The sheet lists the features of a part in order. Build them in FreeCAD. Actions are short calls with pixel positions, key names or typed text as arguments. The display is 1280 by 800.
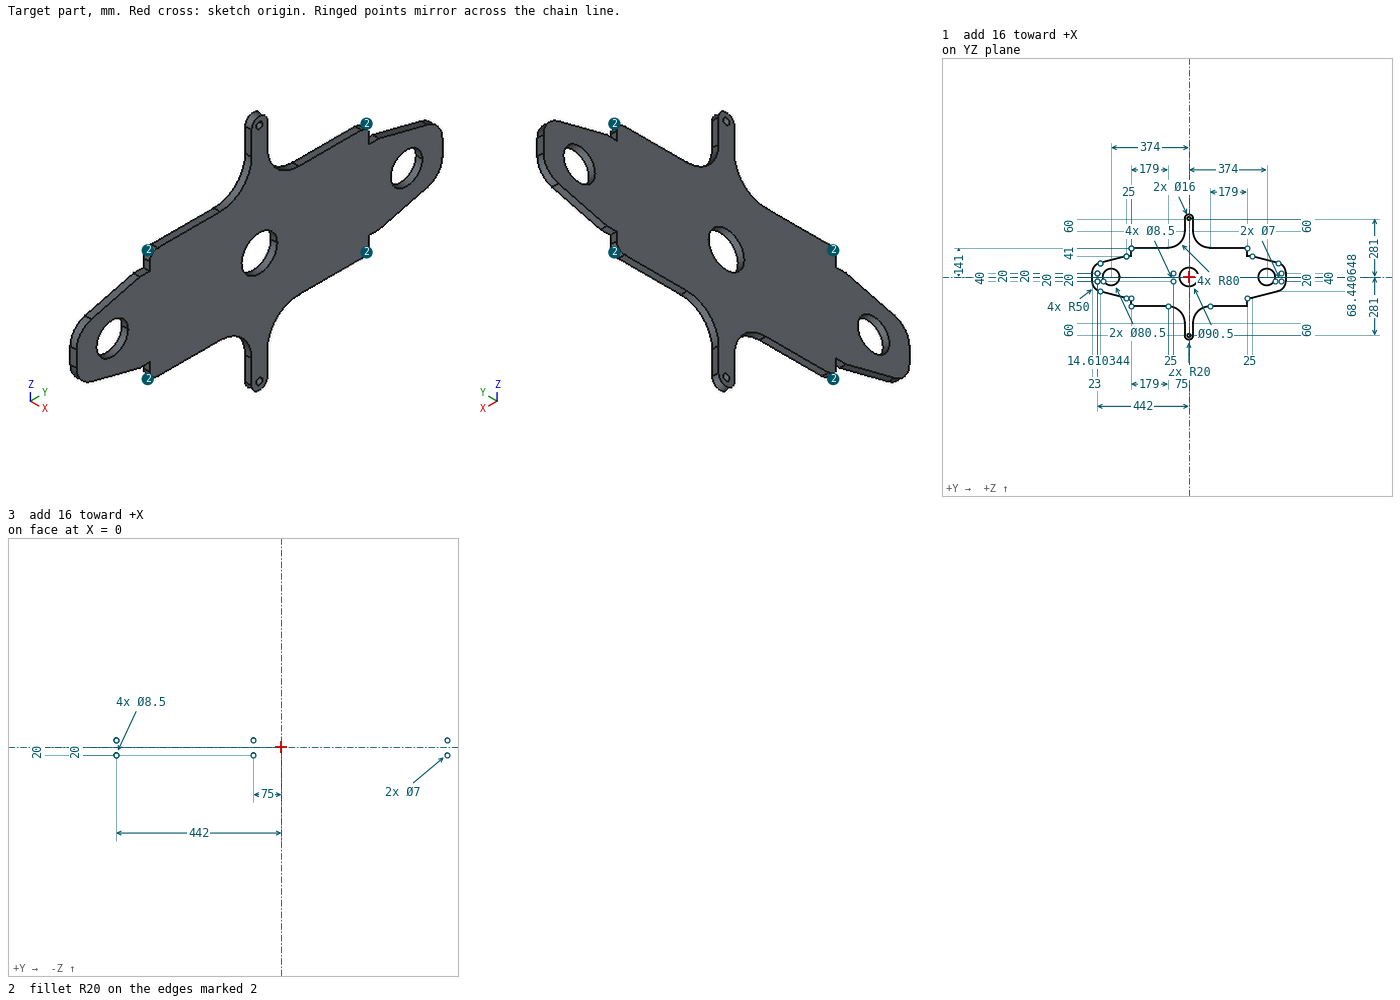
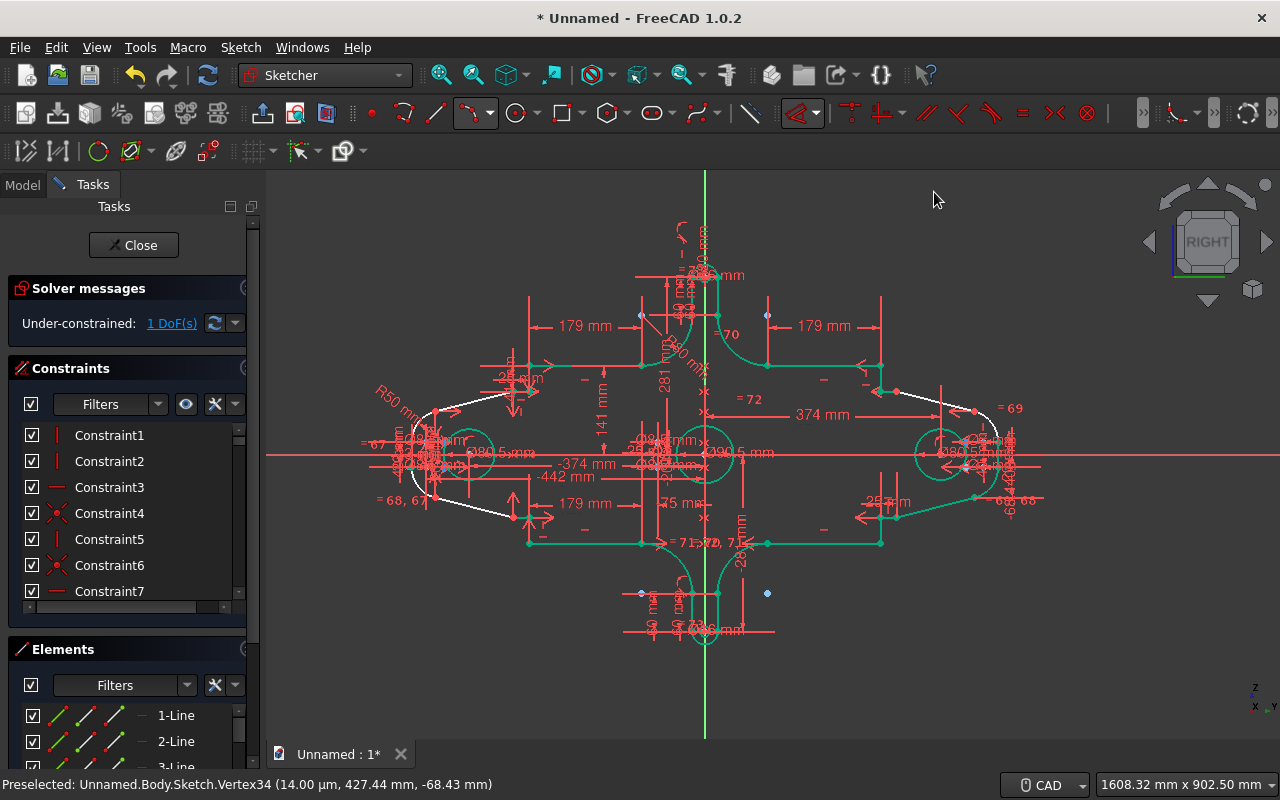
scroll(435, 498, up, 8)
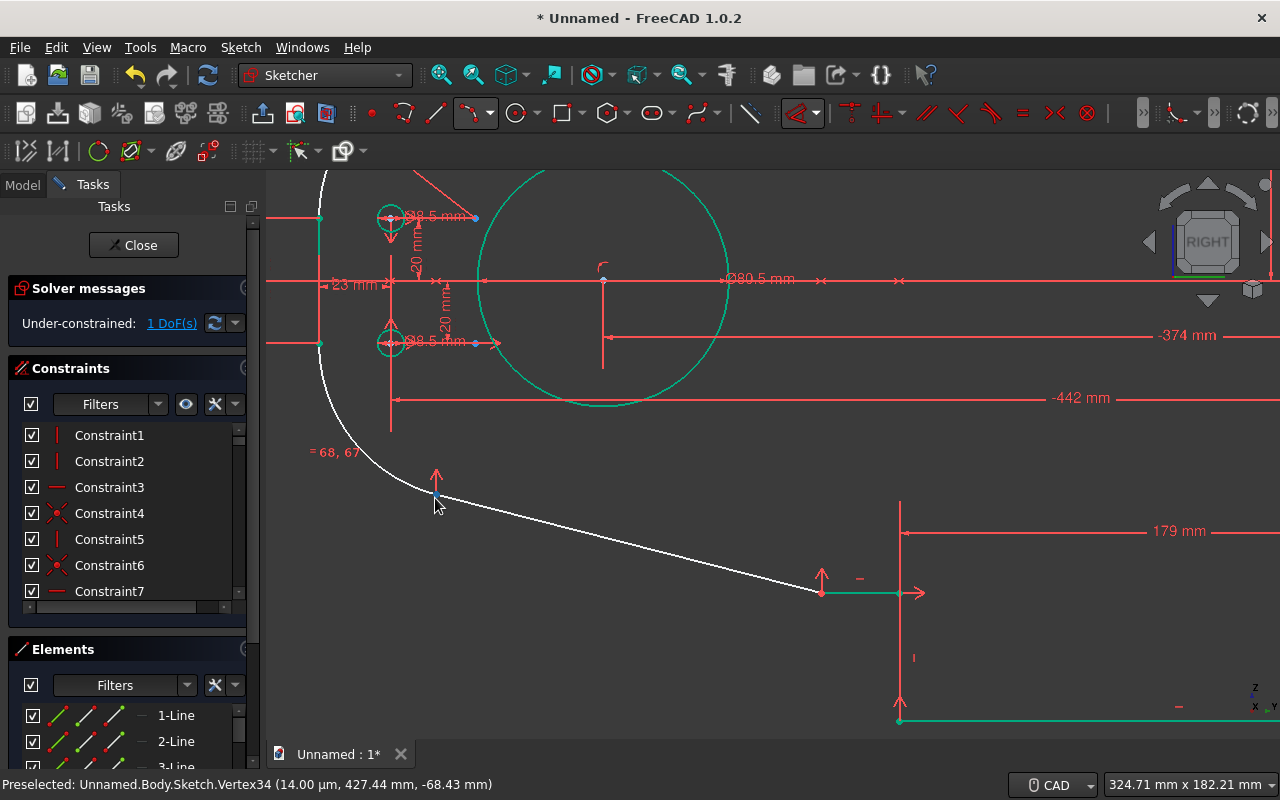
click(436, 495)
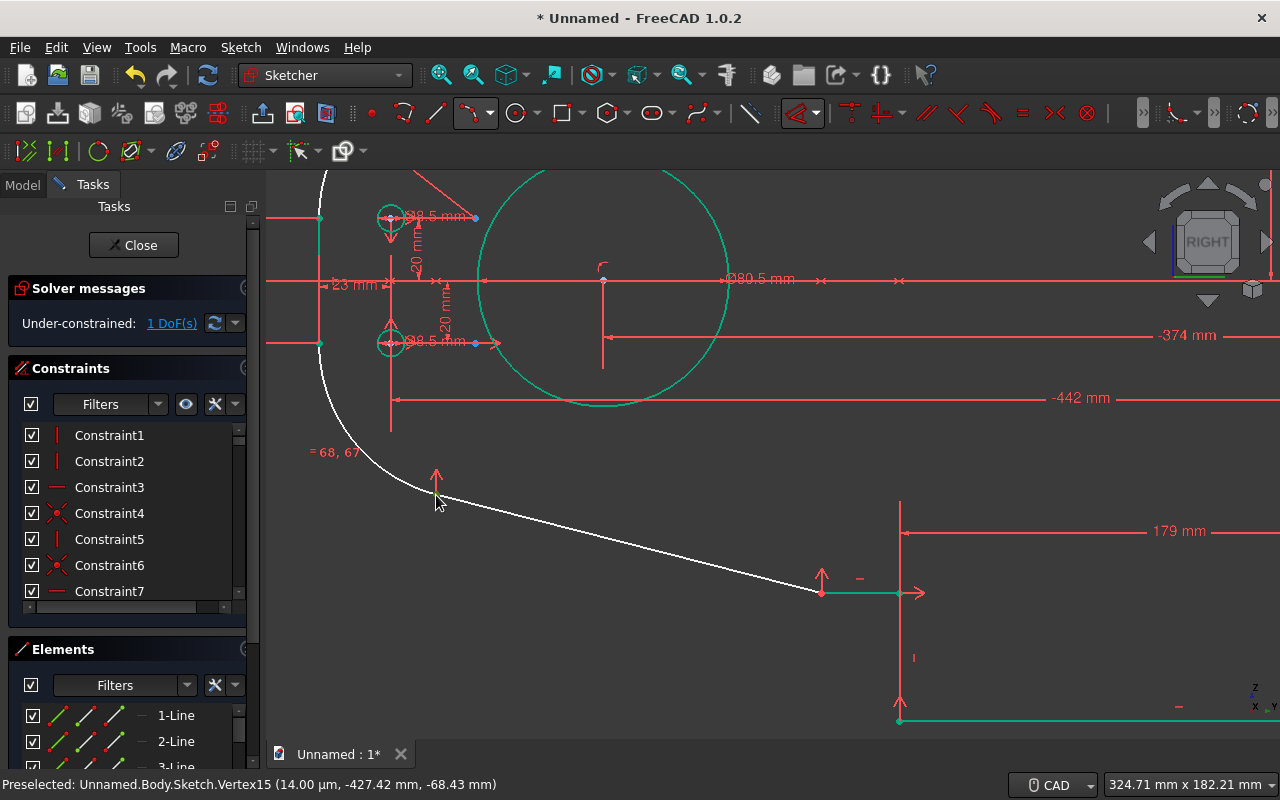
click(391, 343)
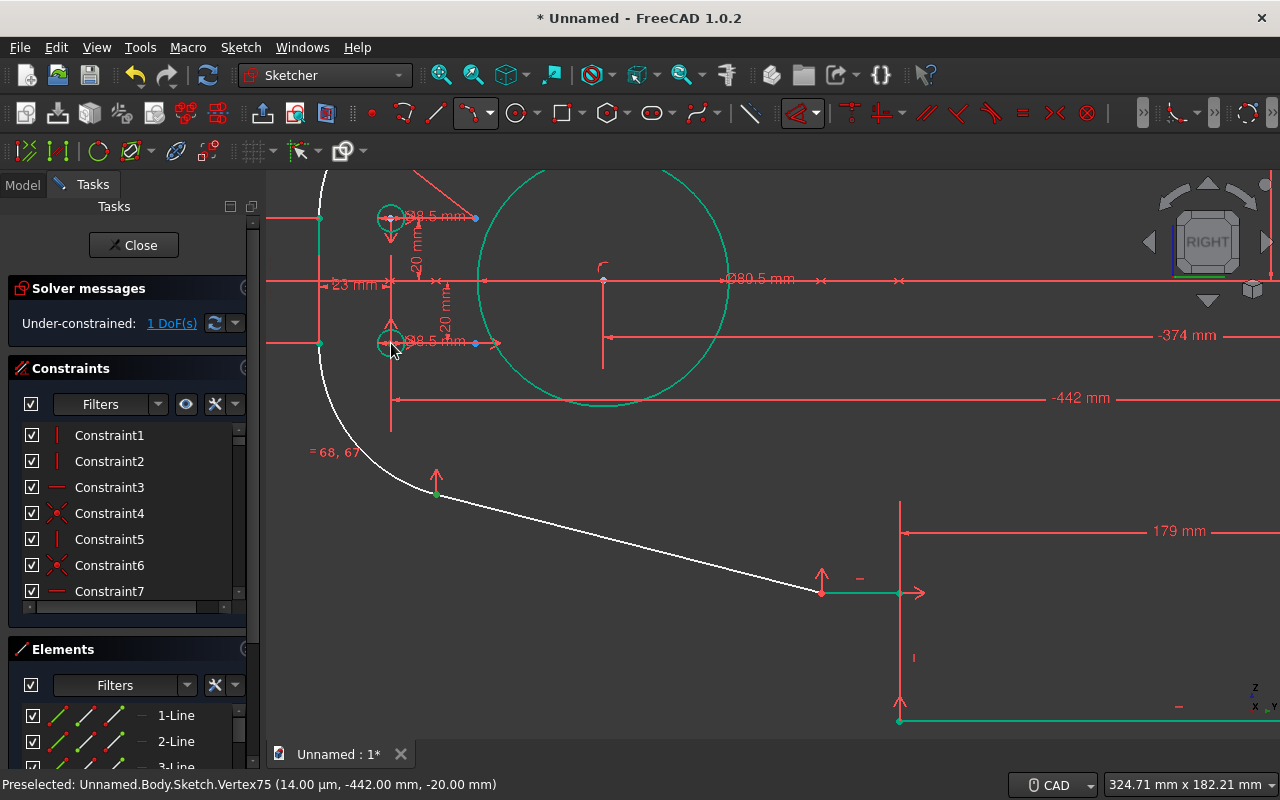
click(818, 114)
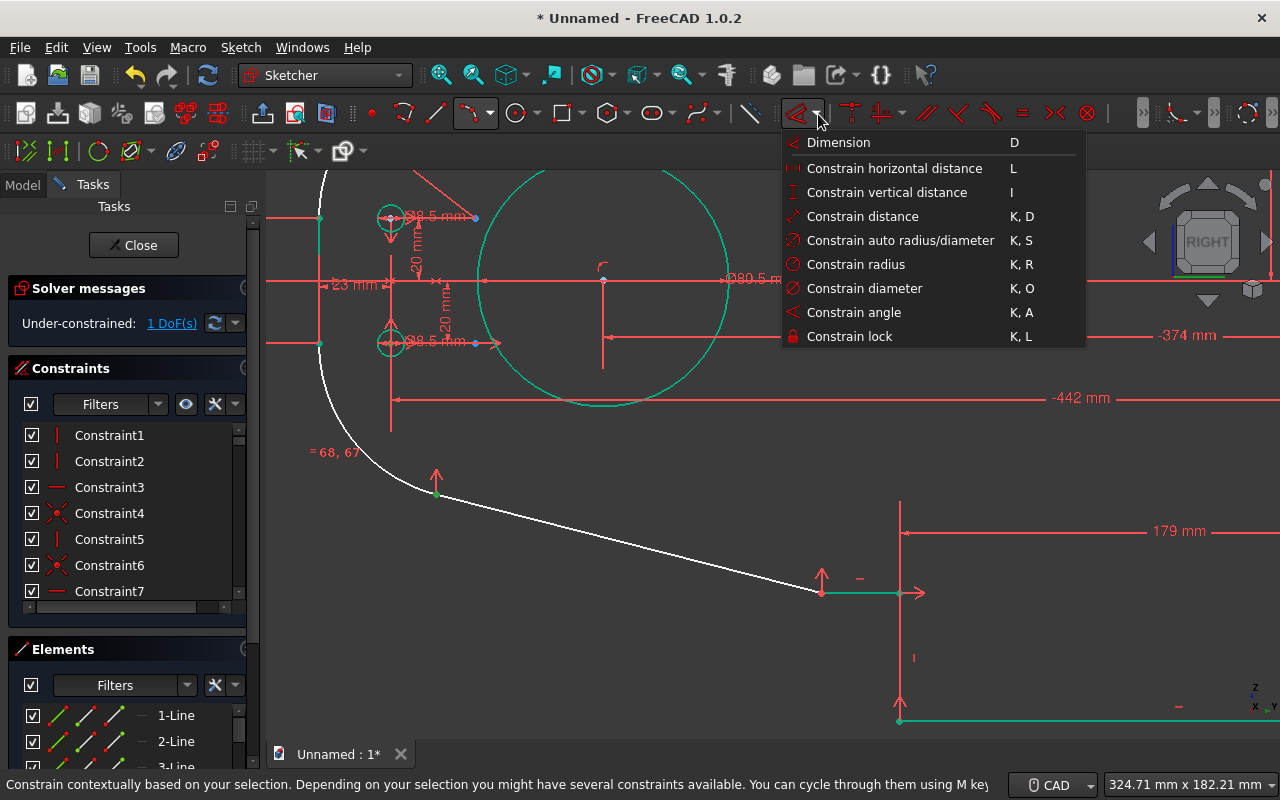
click(934, 168)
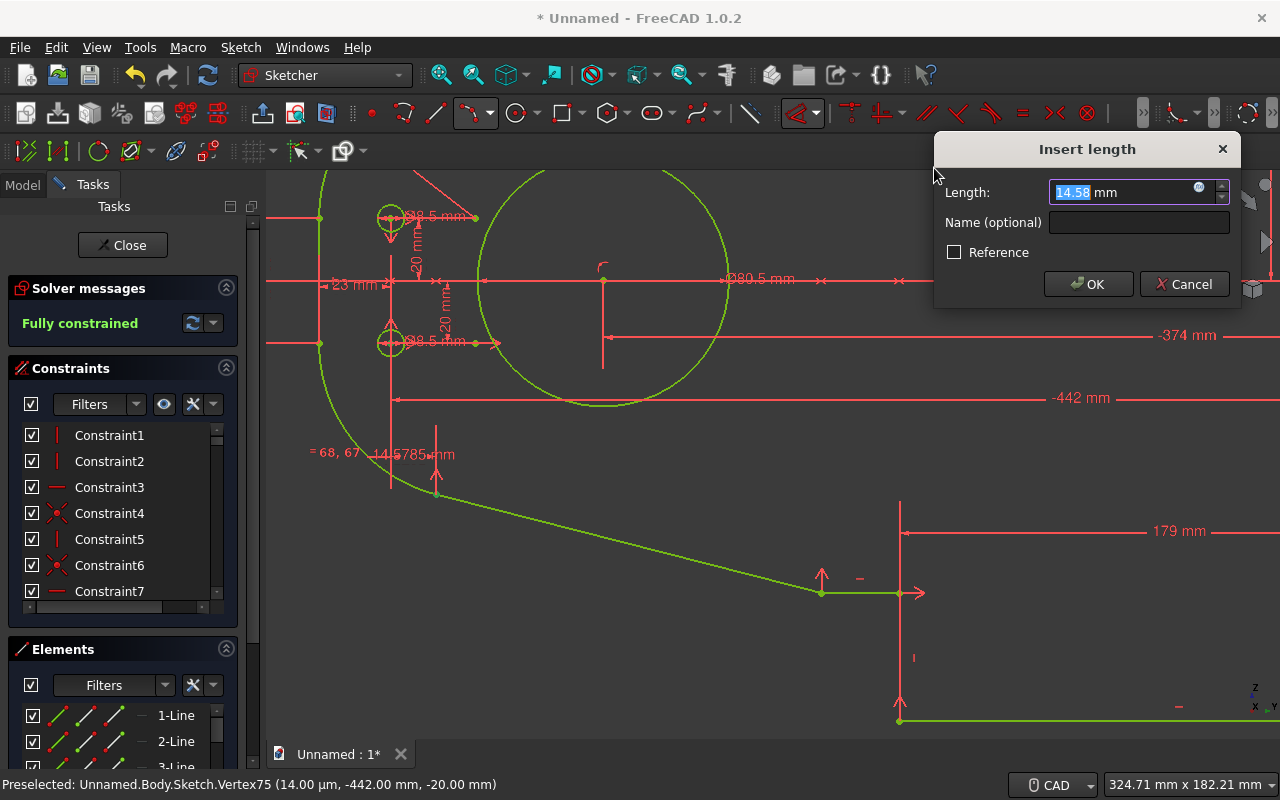
text(14.610344)
key(Return)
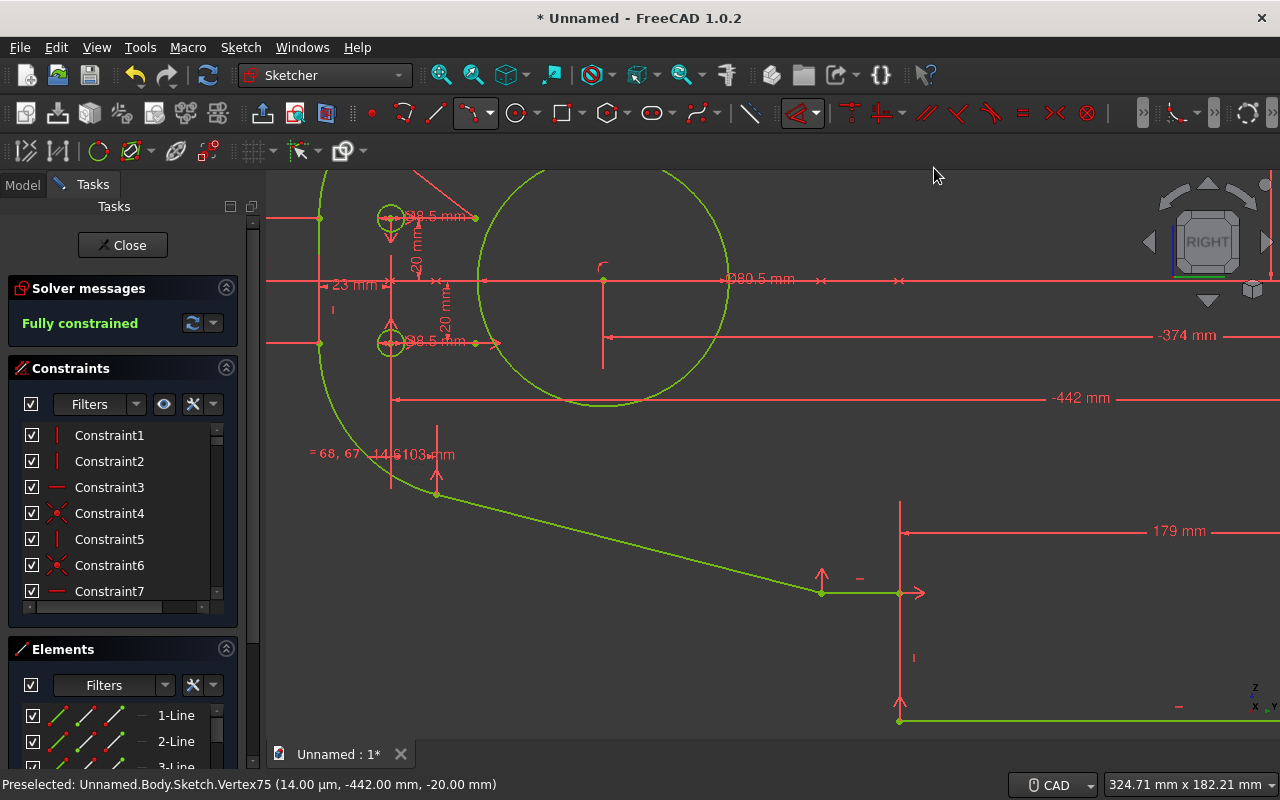
click(123, 245)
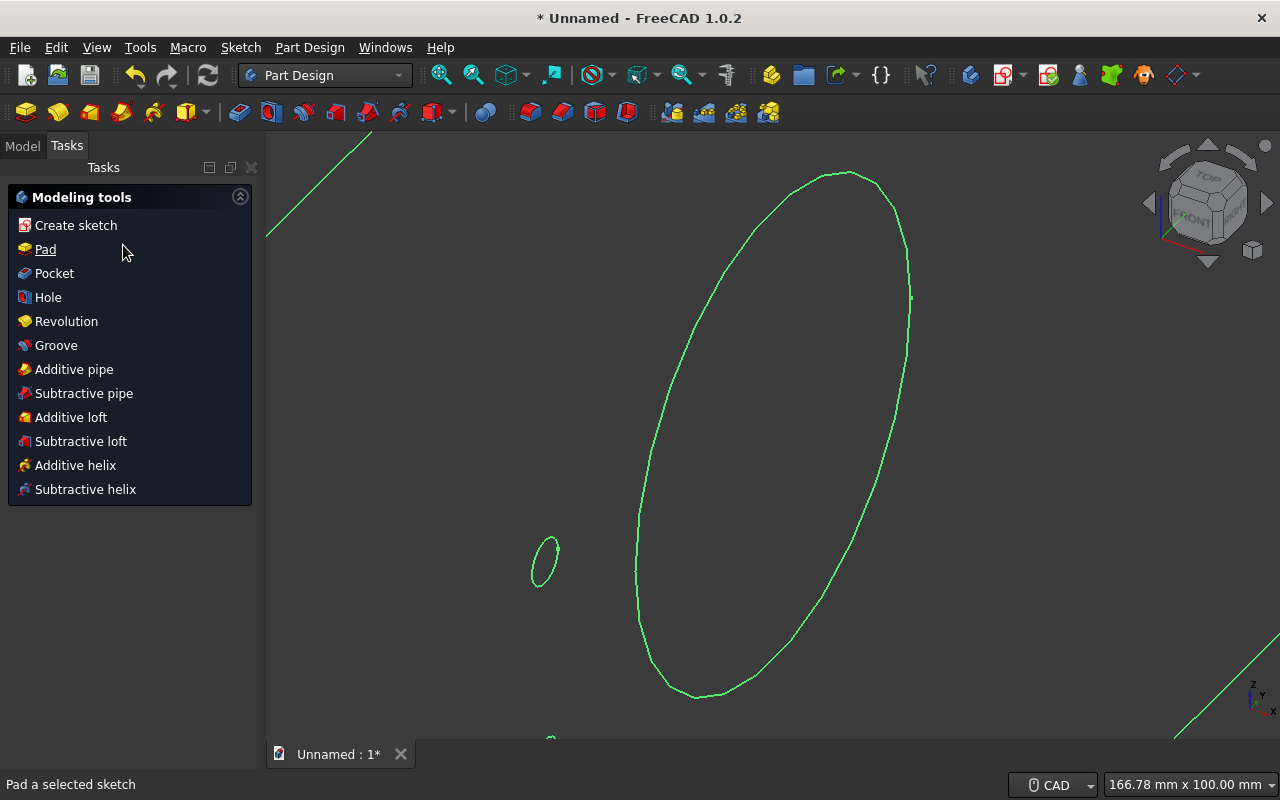
click(26, 112)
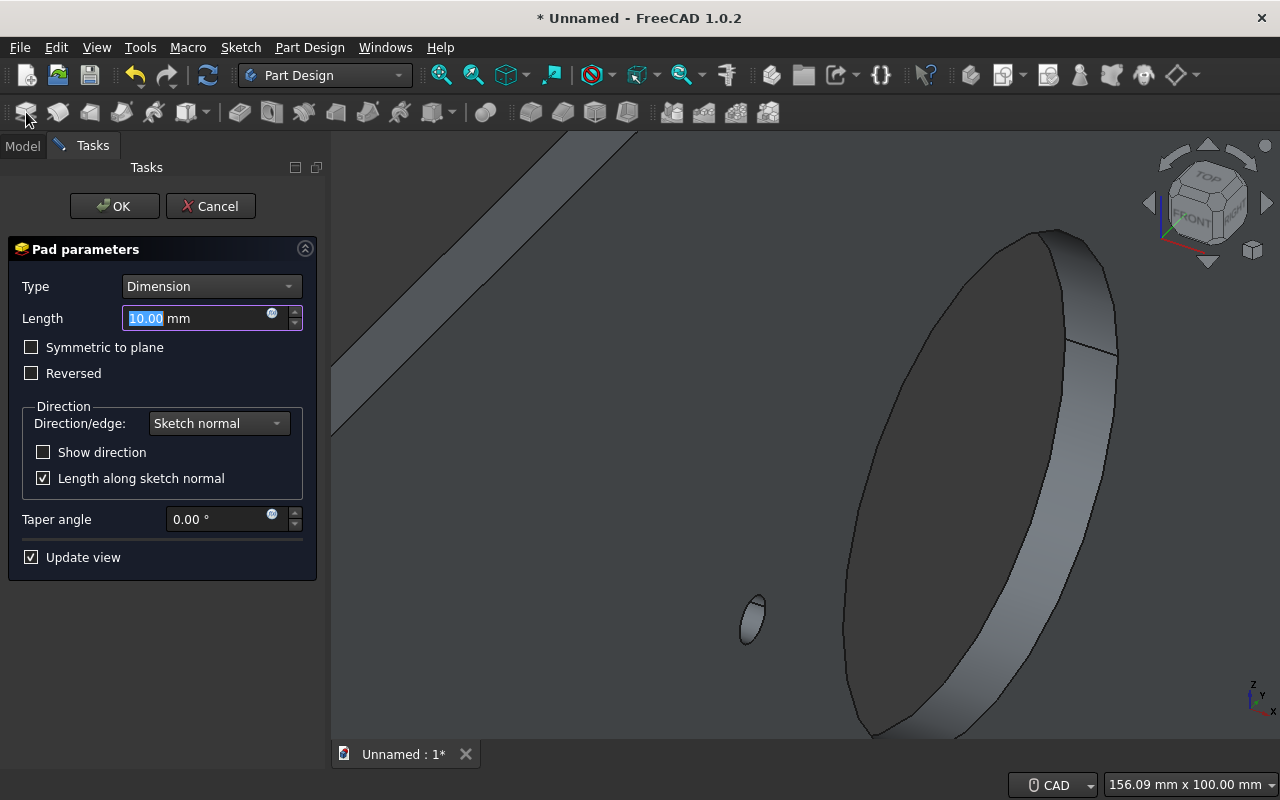
text(16)
key(Tab)